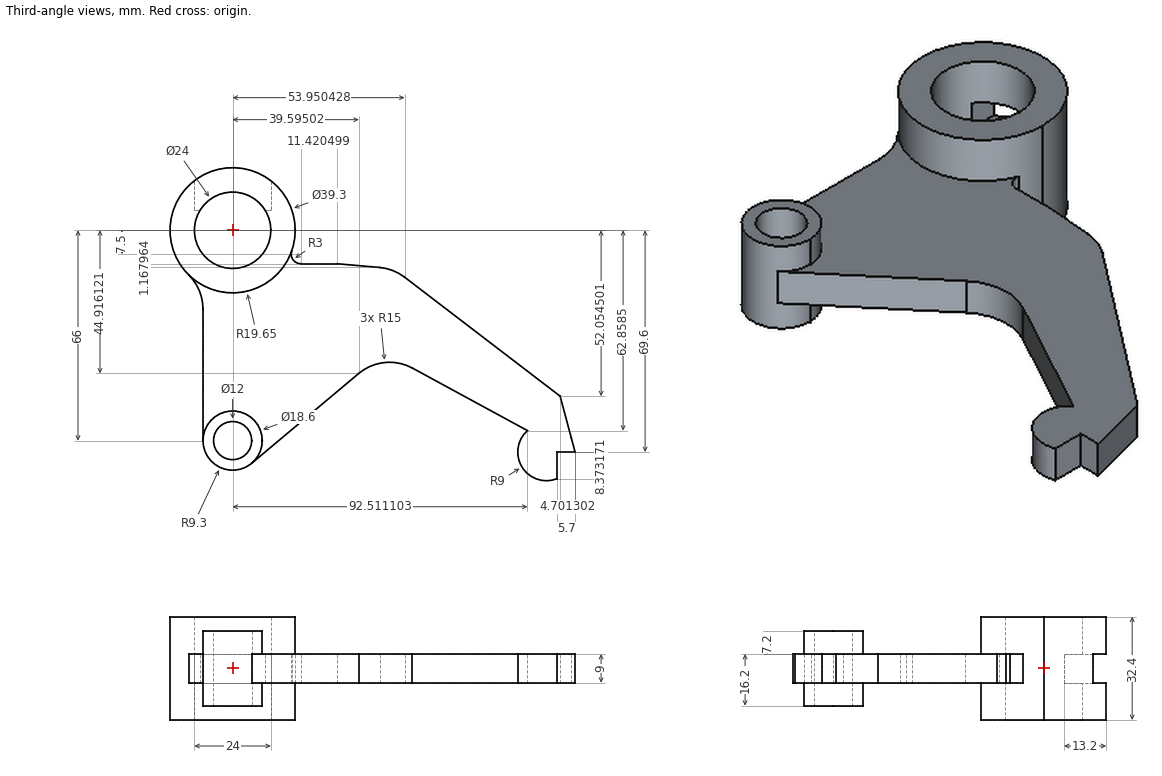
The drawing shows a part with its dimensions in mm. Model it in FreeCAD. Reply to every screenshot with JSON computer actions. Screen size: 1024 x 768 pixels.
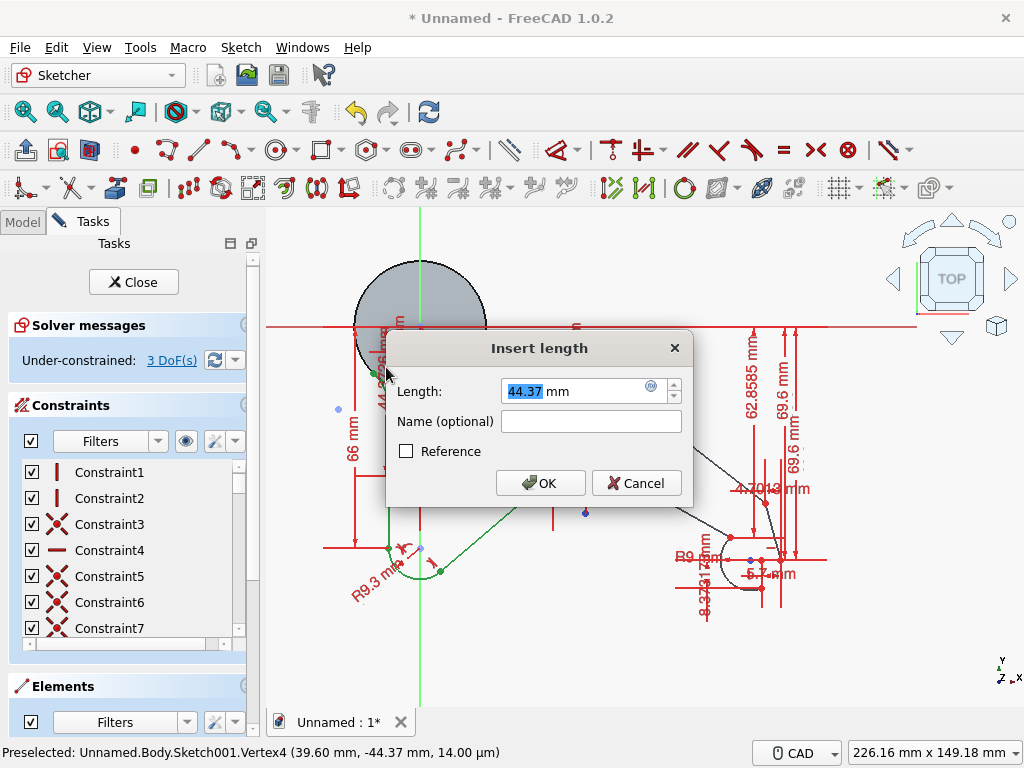
{"action": "type", "text": "44.916121"}
{"action": "key", "text": "Return"}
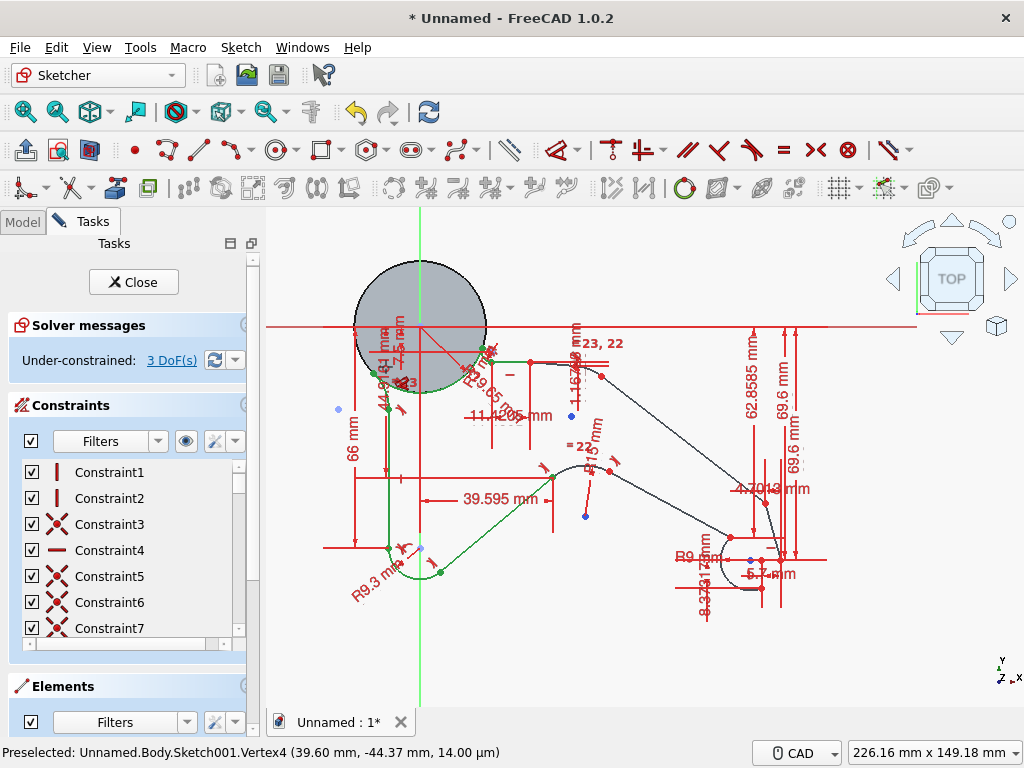
{"action": "left_click", "coordinate": [731, 538]}
{"action": "left_click", "coordinate": [575, 293]}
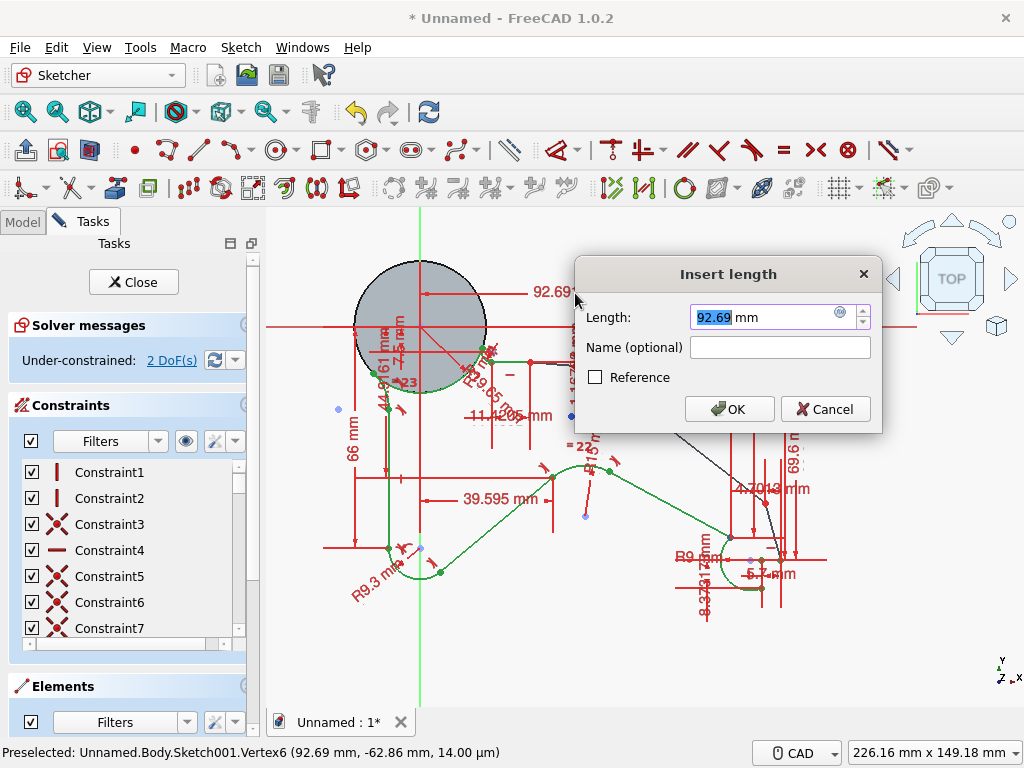
{"action": "type", "text": "92.511103"}
{"action": "key", "text": "Return"}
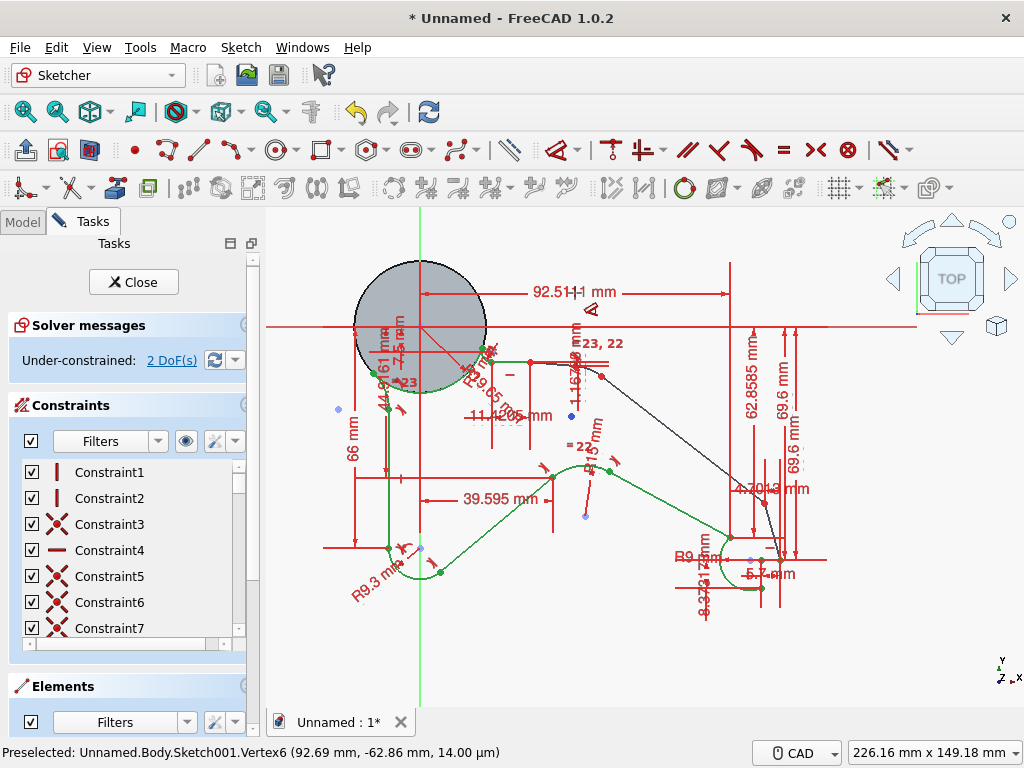
{"action": "left_click", "coordinate": [765, 503]}
{"action": "left_click", "coordinate": [799, 415]}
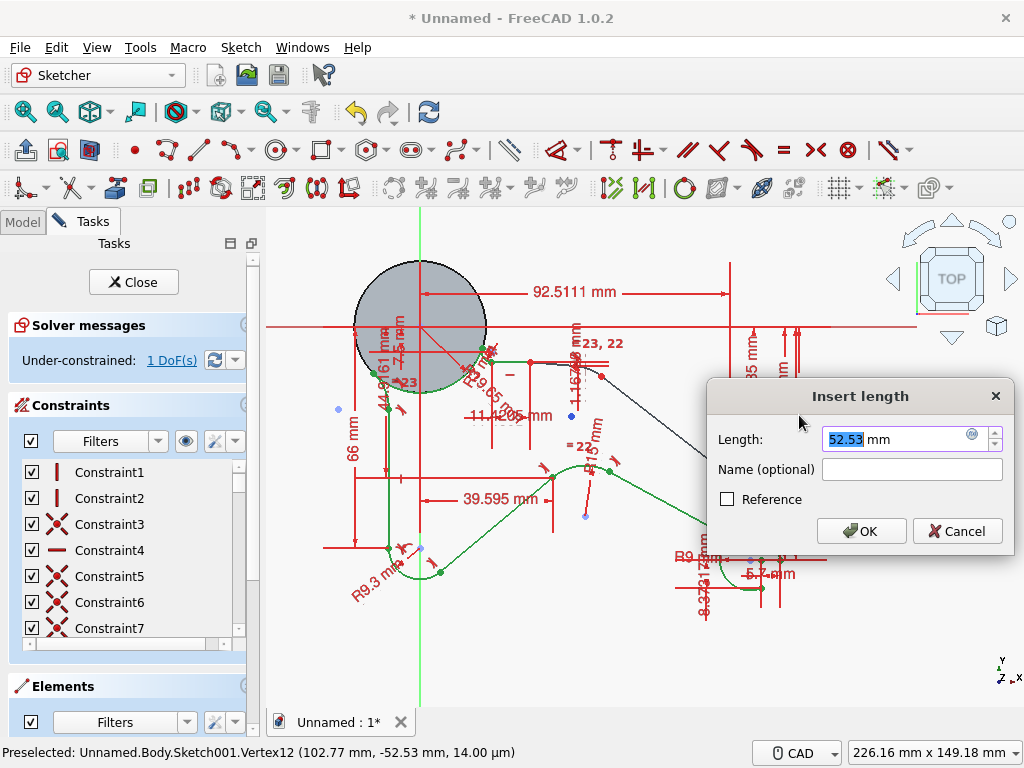
{"action": "type", "text": "52.054501"}
{"action": "key", "text": "Return"}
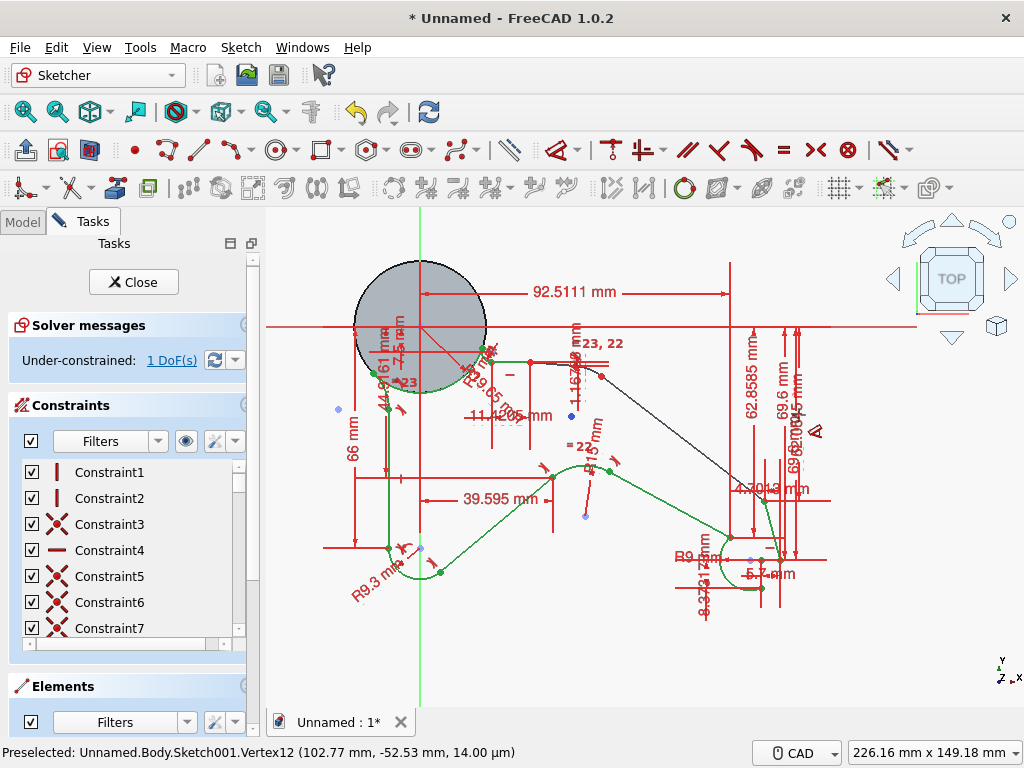
{"action": "left_click", "coordinate": [602, 376]}
{"action": "left_click", "coordinate": [469, 293]}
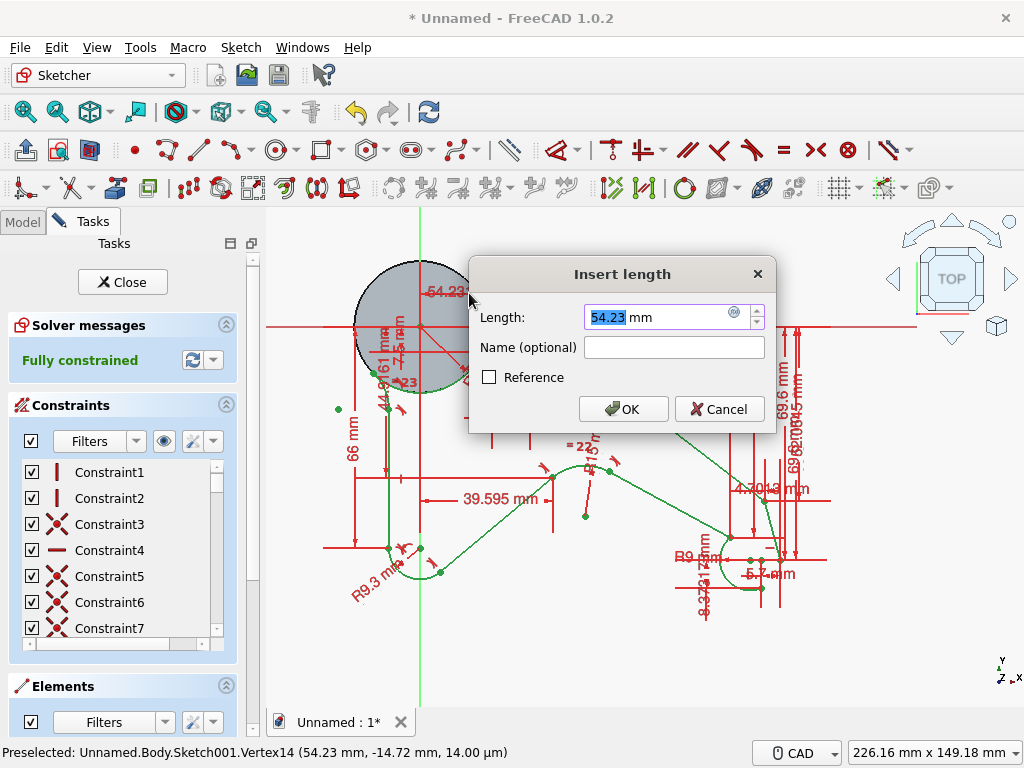
{"action": "type", "text": "53.950428"}
{"action": "key", "text": "Return"}
{"action": "key", "text": "Escape"}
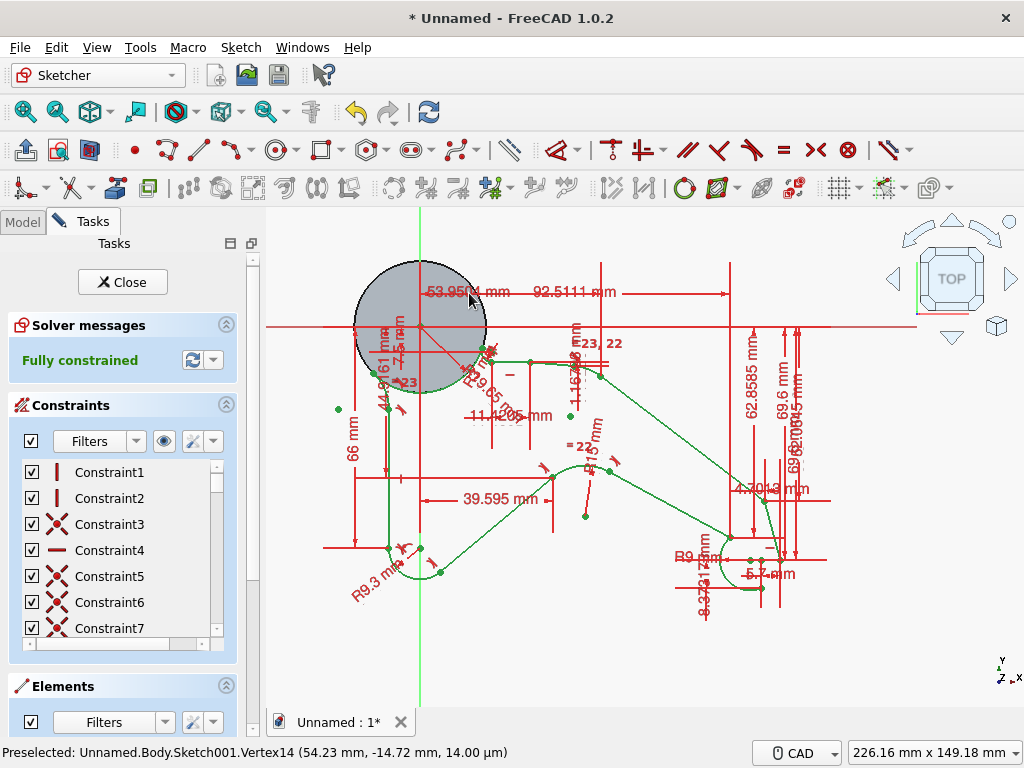
{"action": "left_click", "coordinate": [123, 282]}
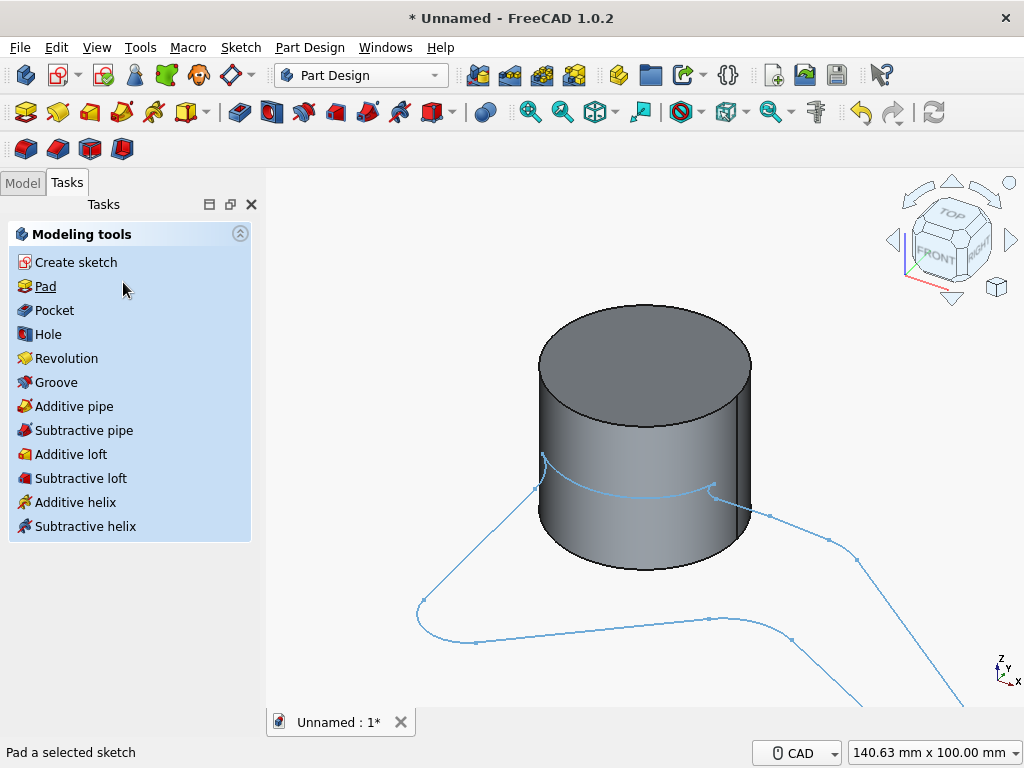
{"action": "left_click", "coordinate": [26, 112]}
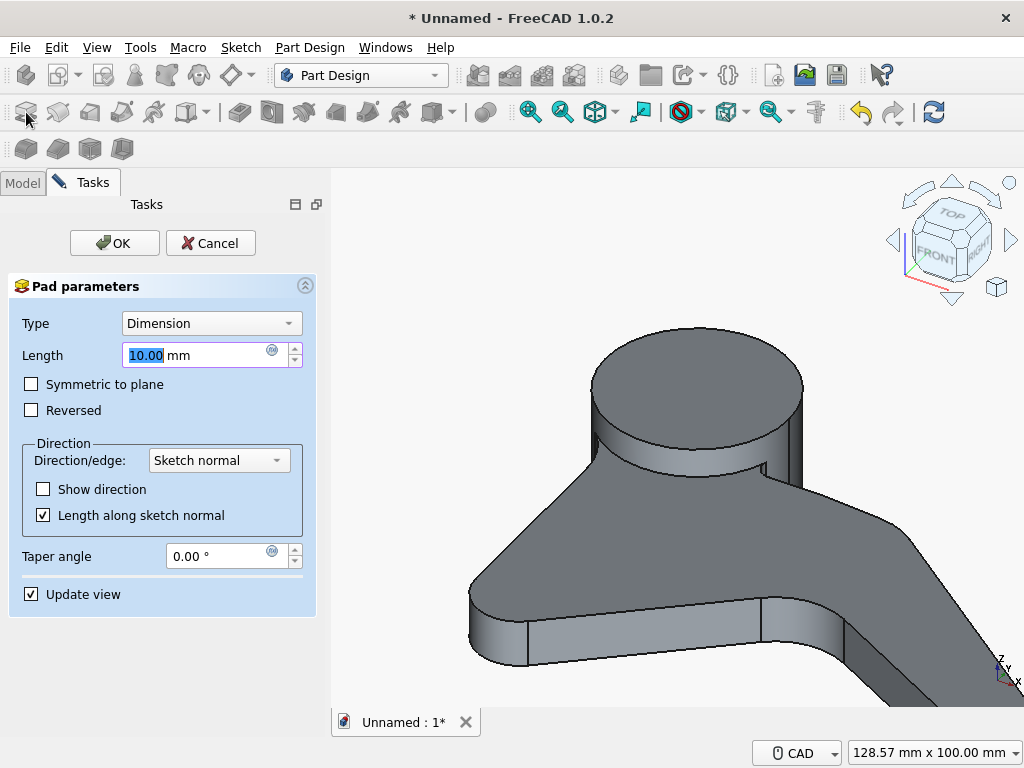
{"action": "type", "text": "9"}
{"action": "key", "text": "Tab"}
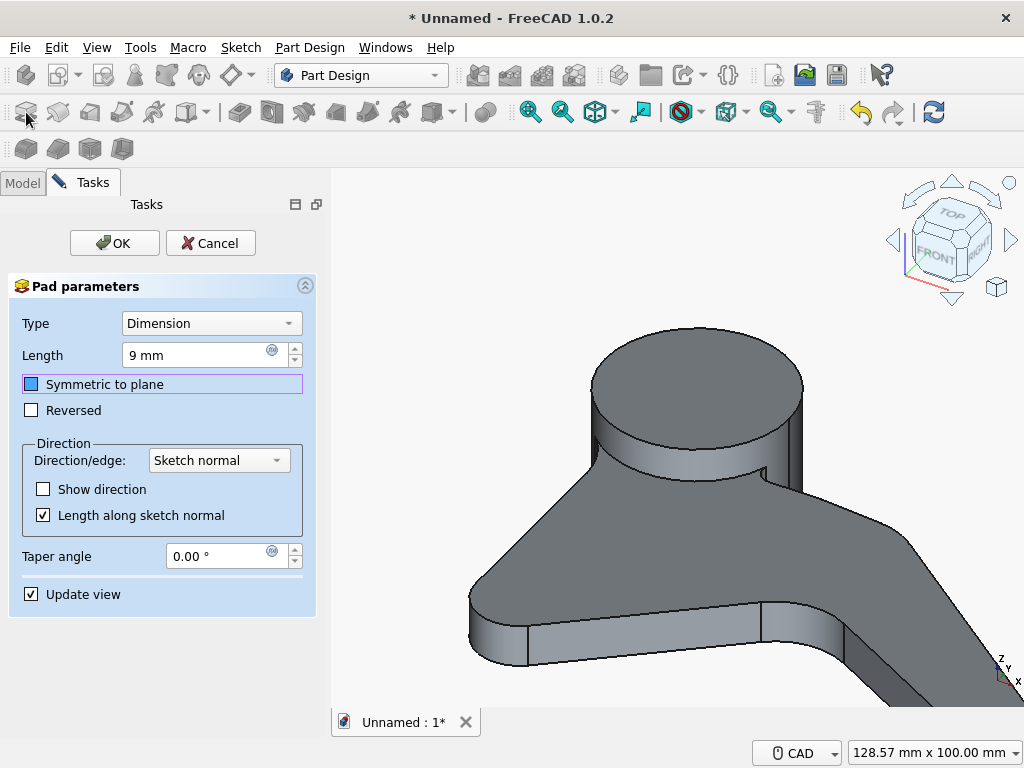
{"action": "left_click", "coordinate": [30, 384]}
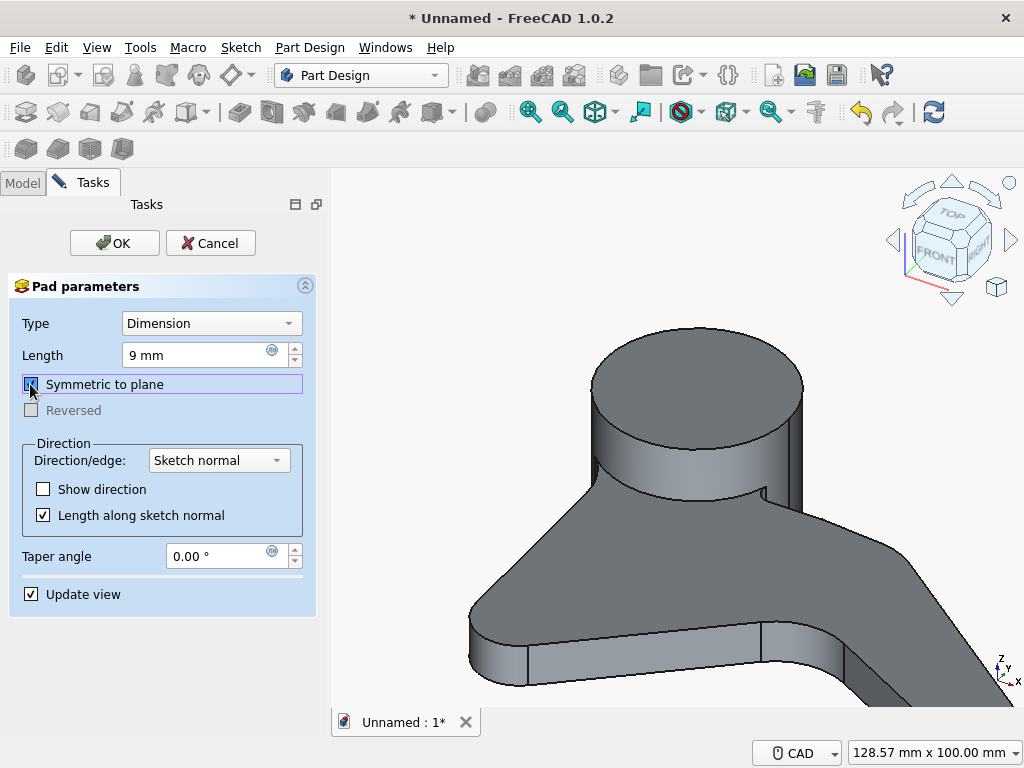
{"action": "left_click", "coordinate": [115, 243]}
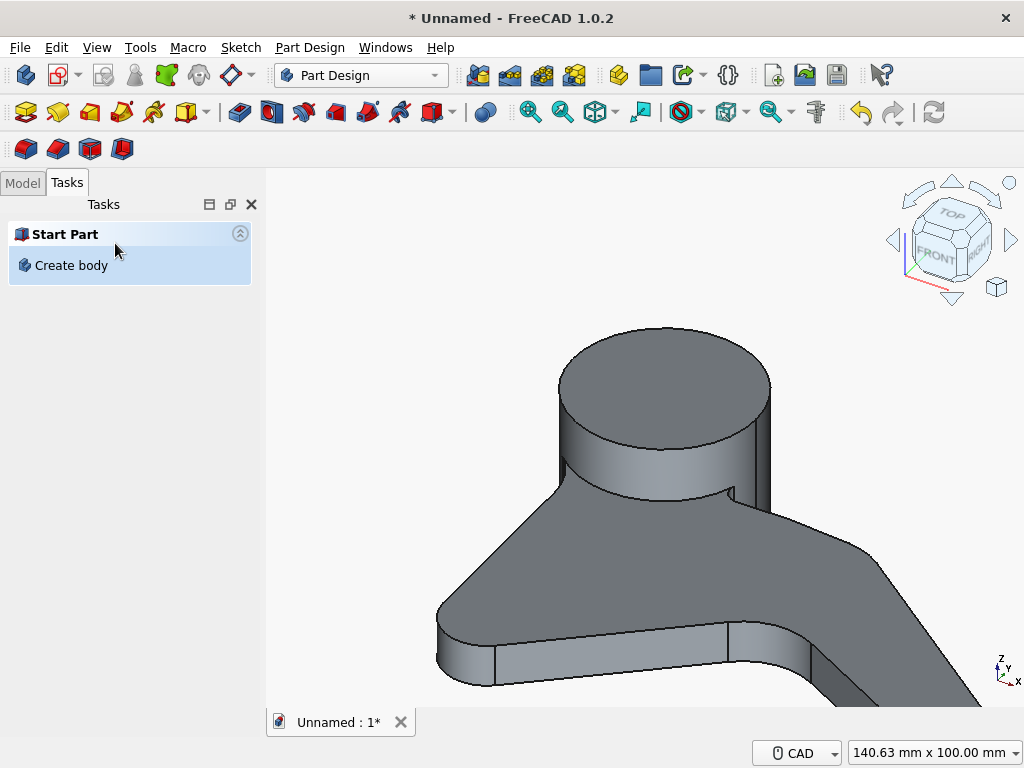
{"action": "left_click", "coordinate": [532, 112]}